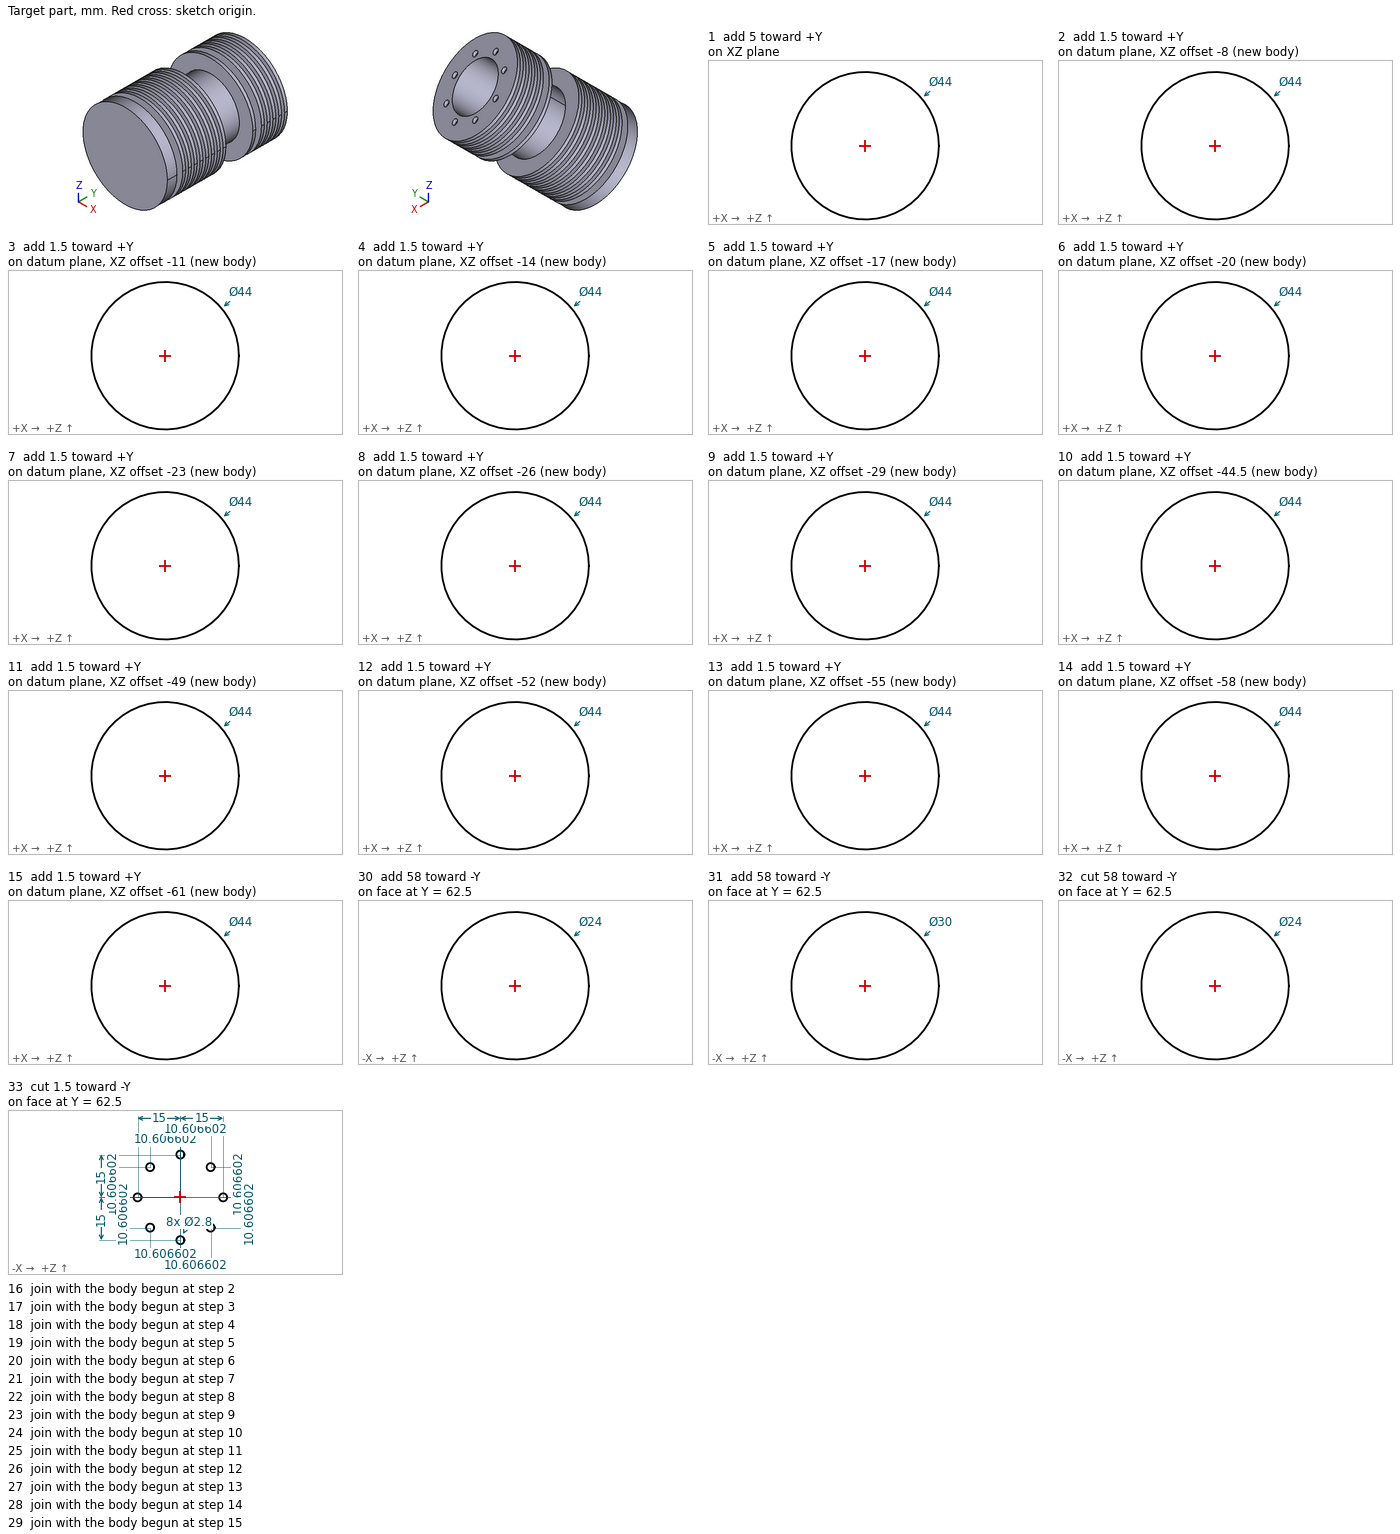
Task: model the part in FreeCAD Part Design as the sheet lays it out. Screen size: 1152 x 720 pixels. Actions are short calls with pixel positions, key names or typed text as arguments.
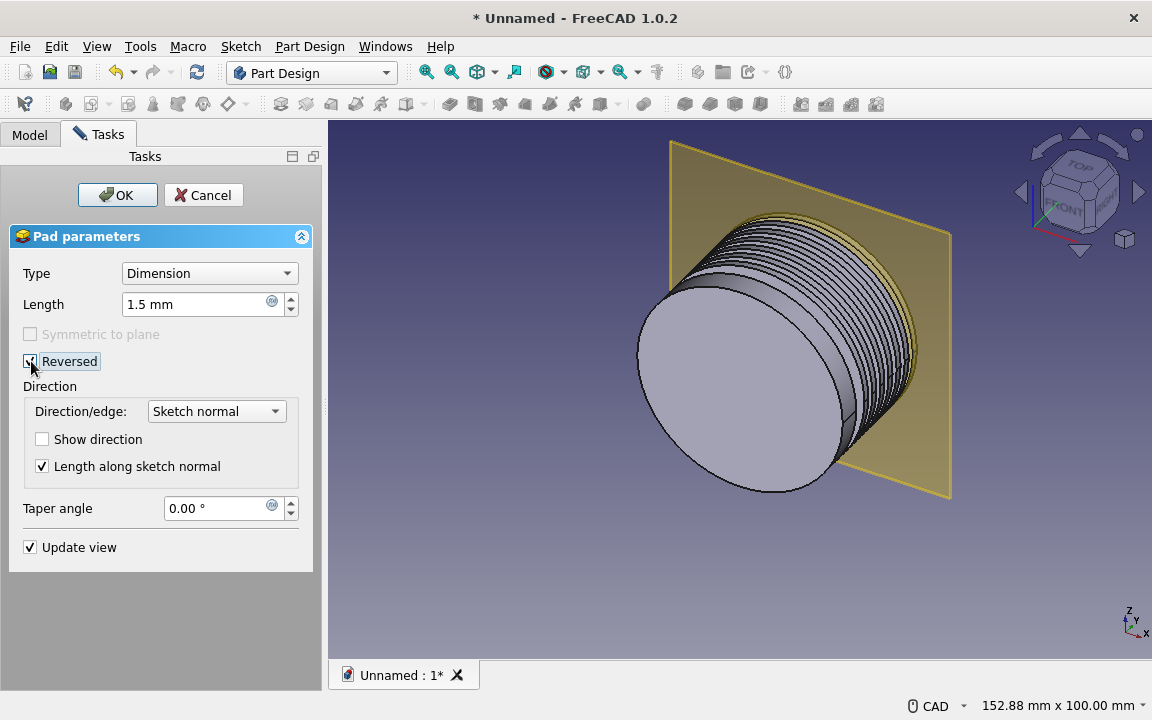
click(118, 195)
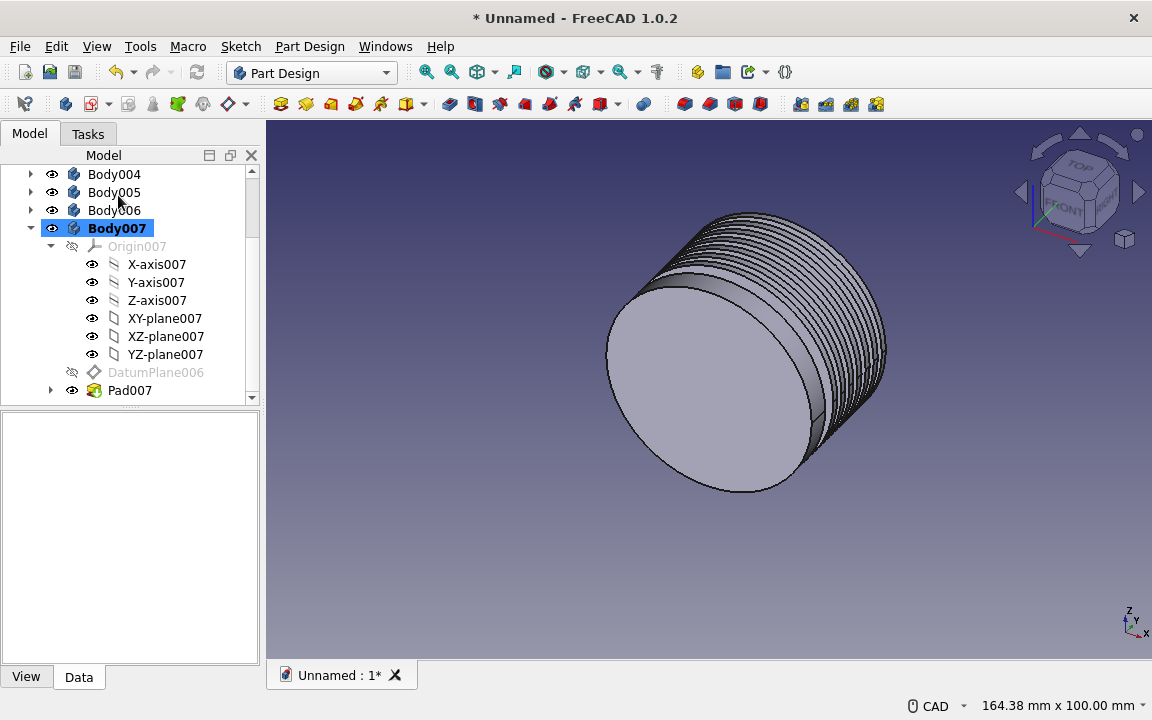
click(66, 104)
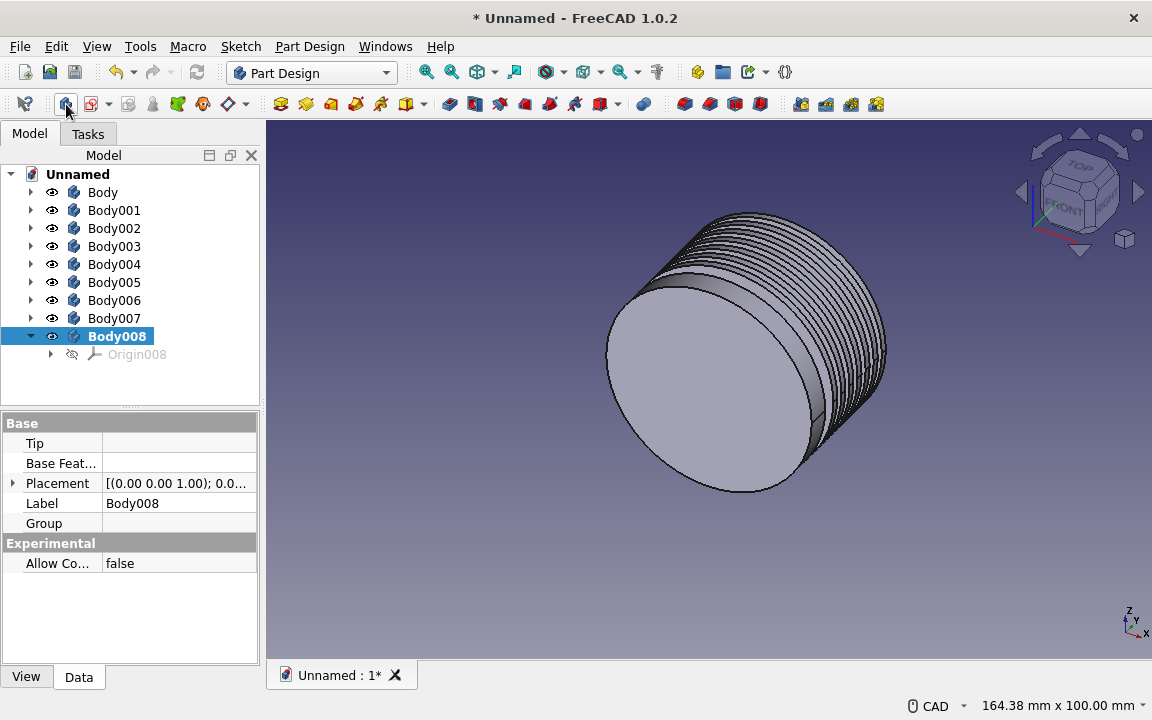
click(51, 354)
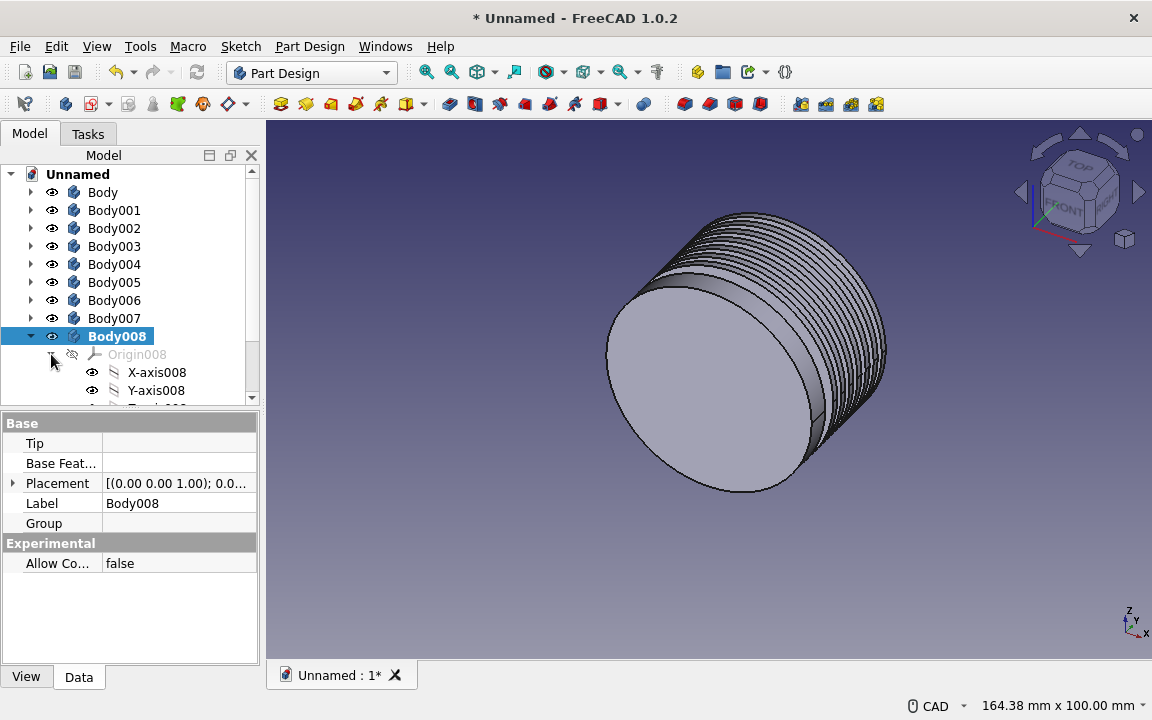
scroll(101, 278, down, 3)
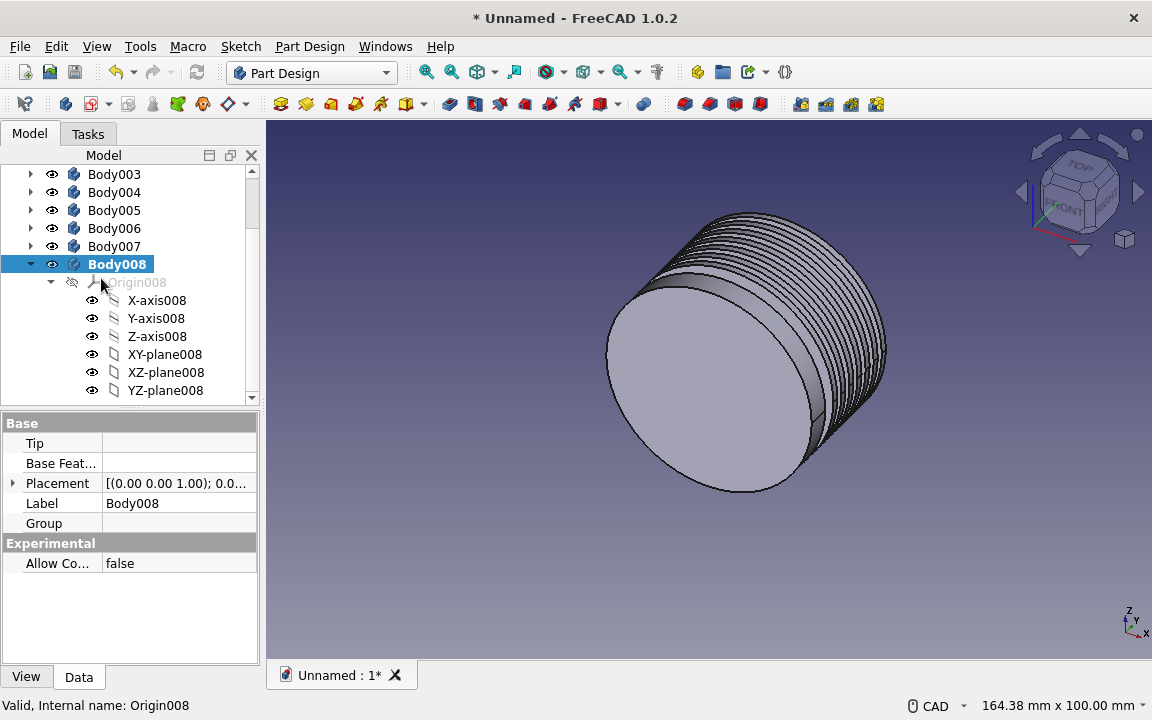
click(137, 372)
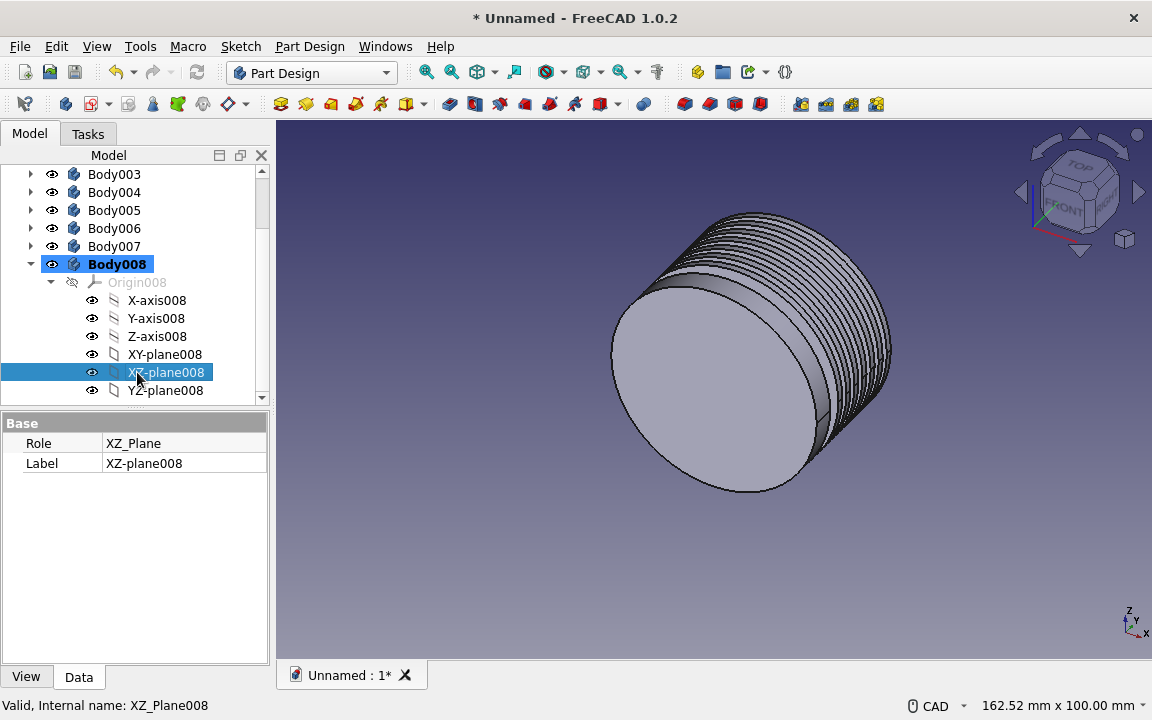
click(228, 104)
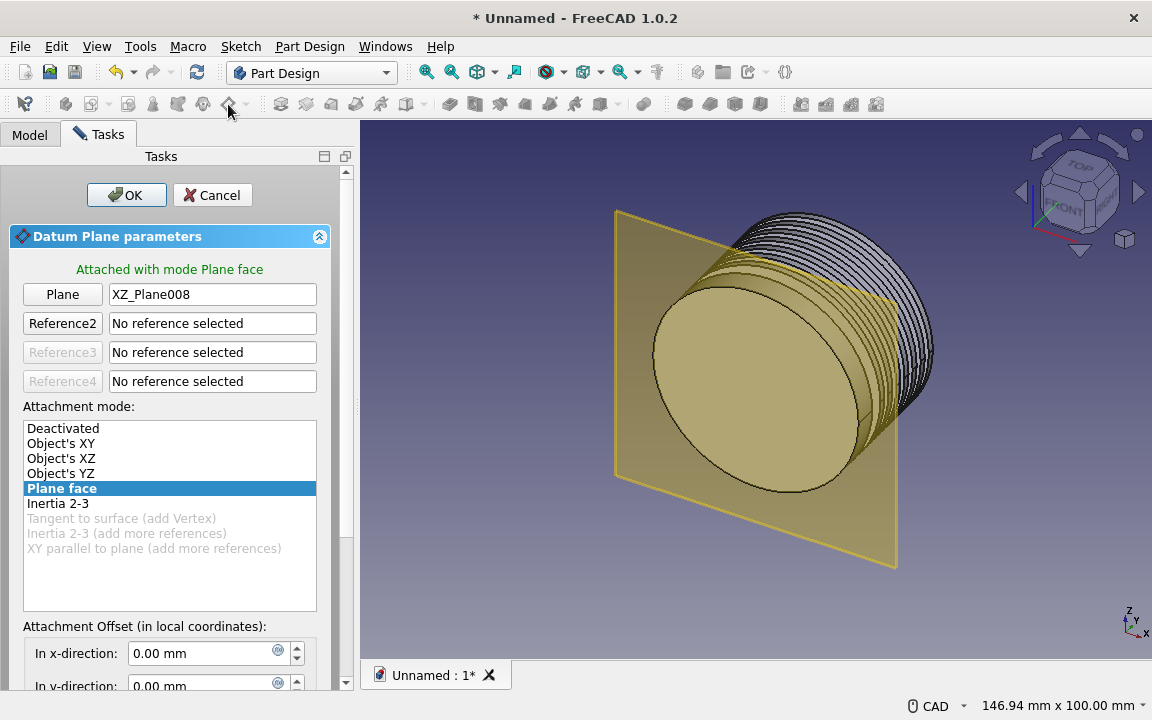
scroll(346, 428, down, 2)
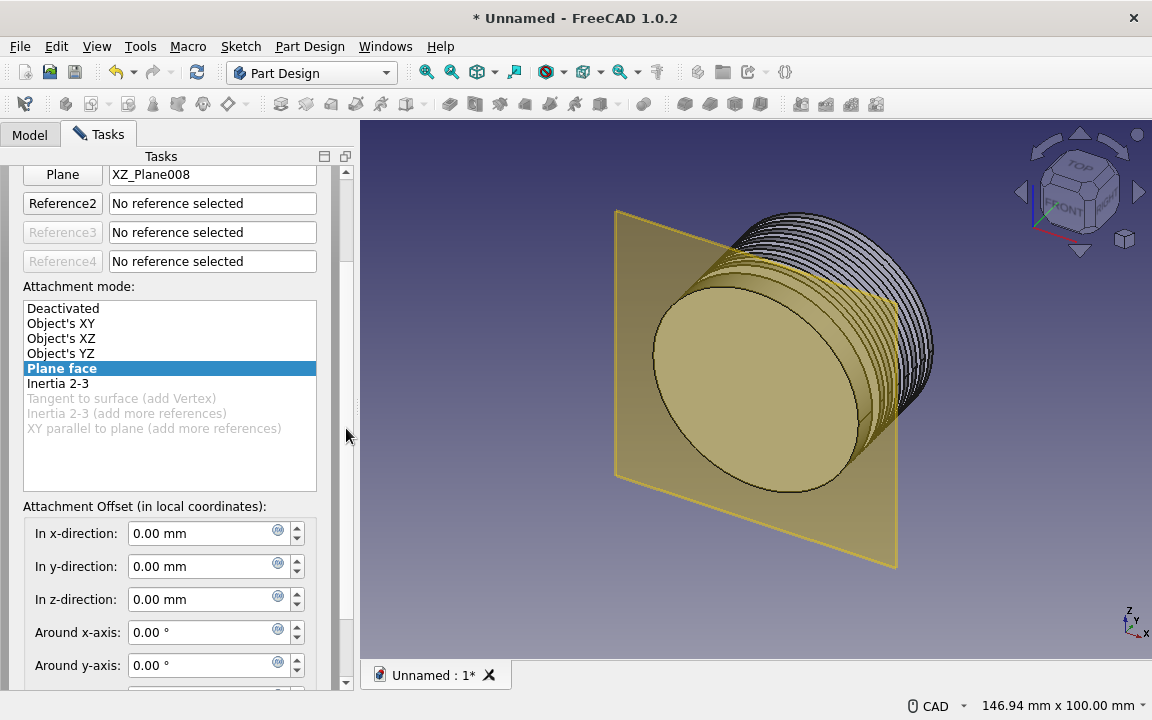
triple_click(210, 600)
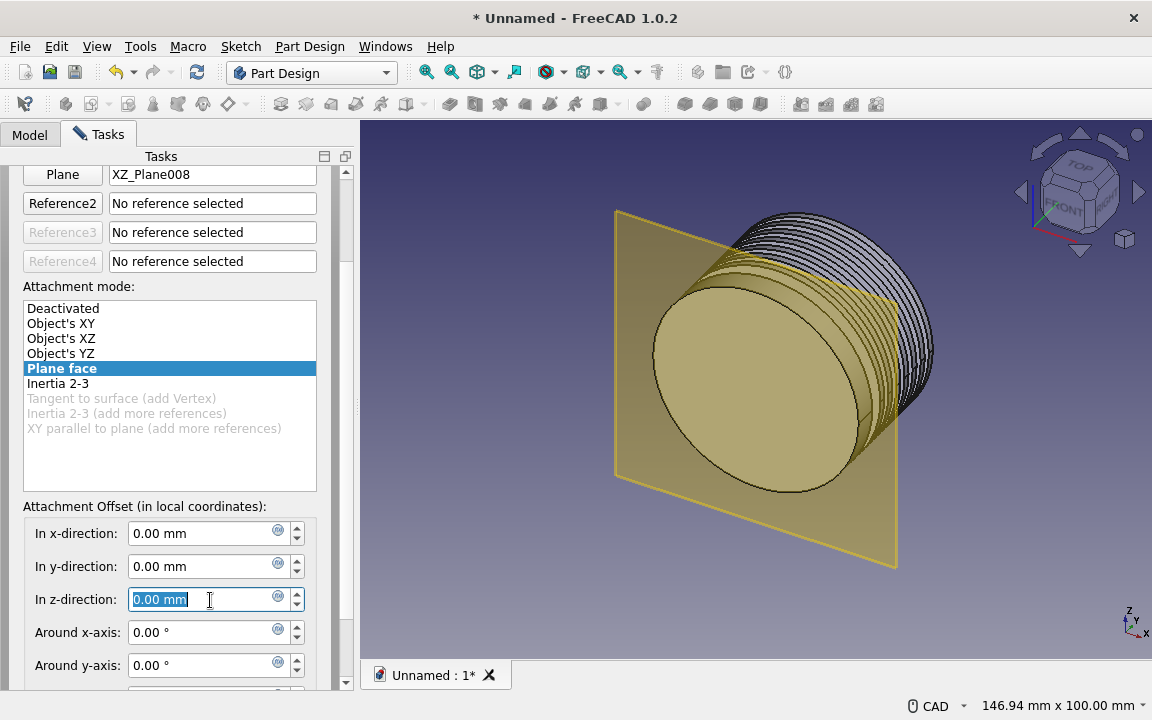
text(-29)
key(Tab)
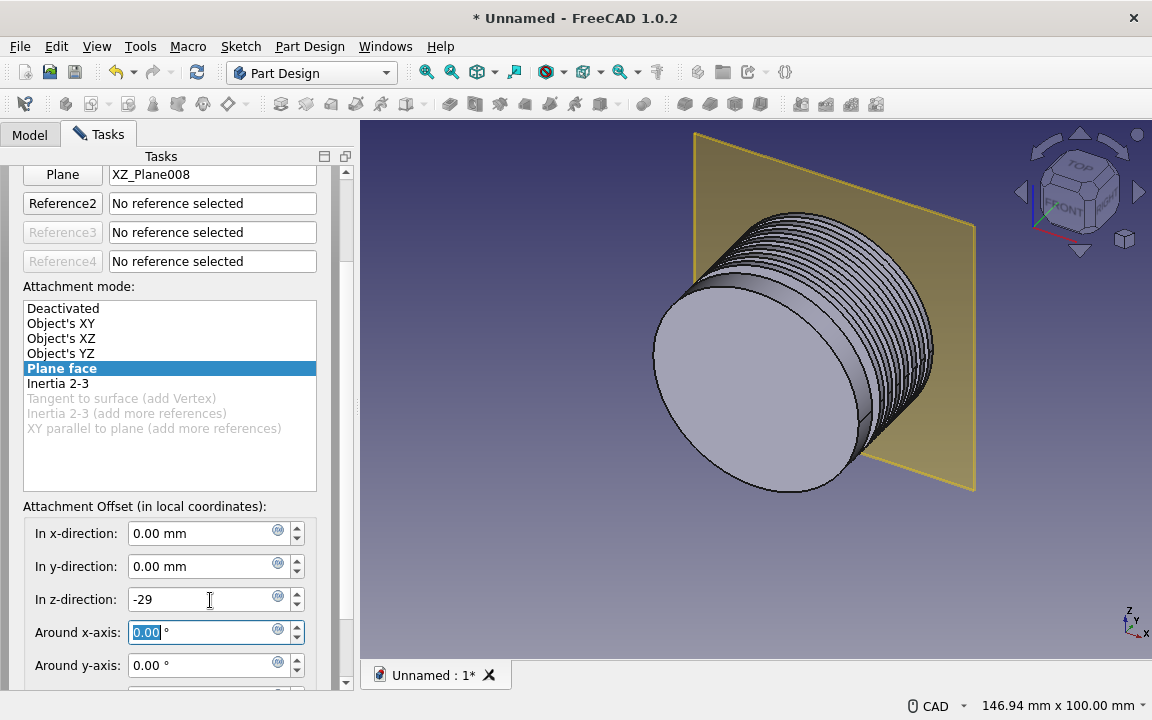
scroll(346, 428, up, 3)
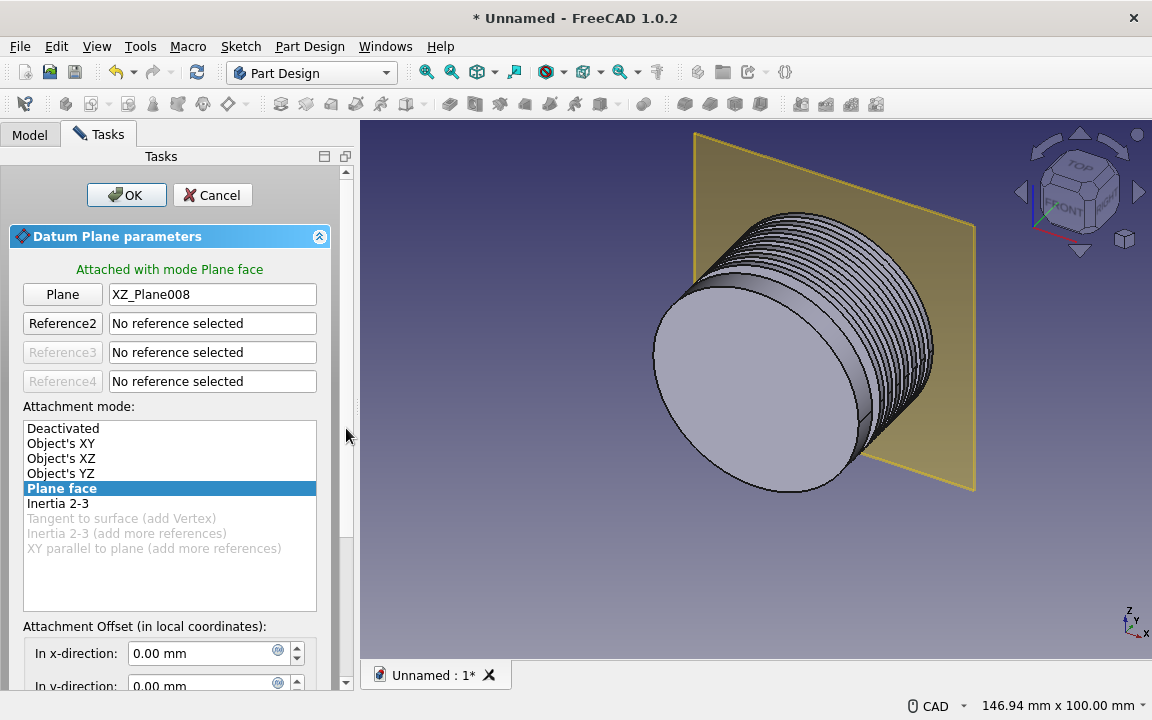
click(127, 195)